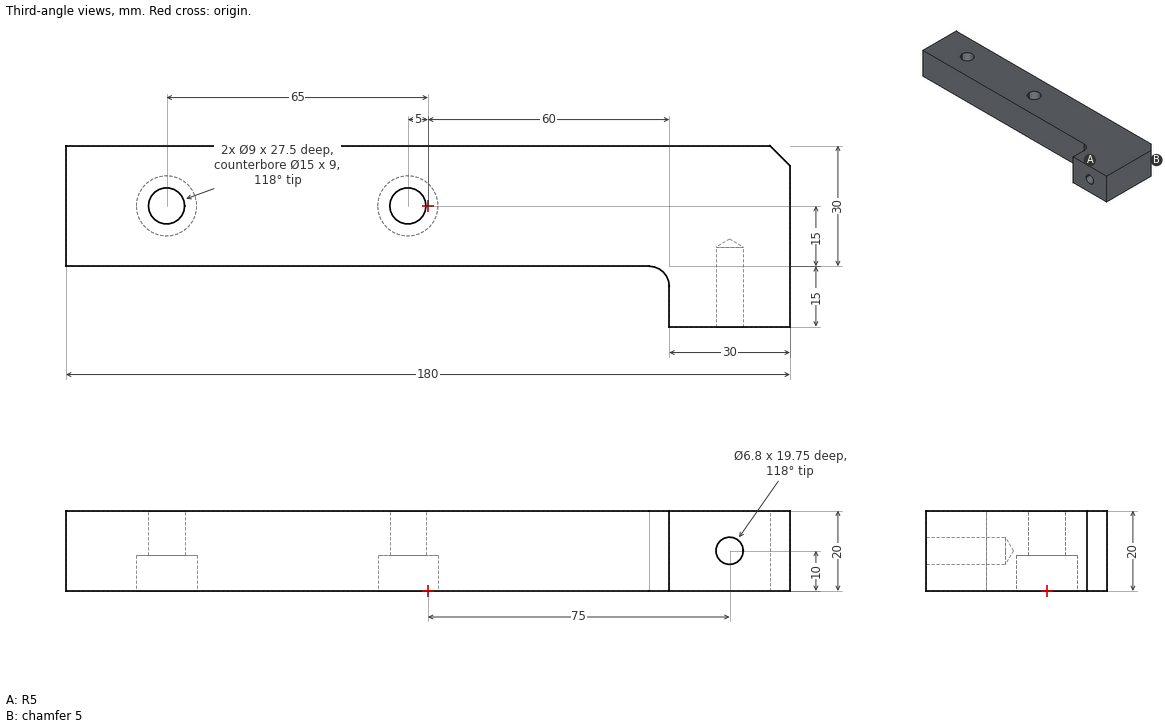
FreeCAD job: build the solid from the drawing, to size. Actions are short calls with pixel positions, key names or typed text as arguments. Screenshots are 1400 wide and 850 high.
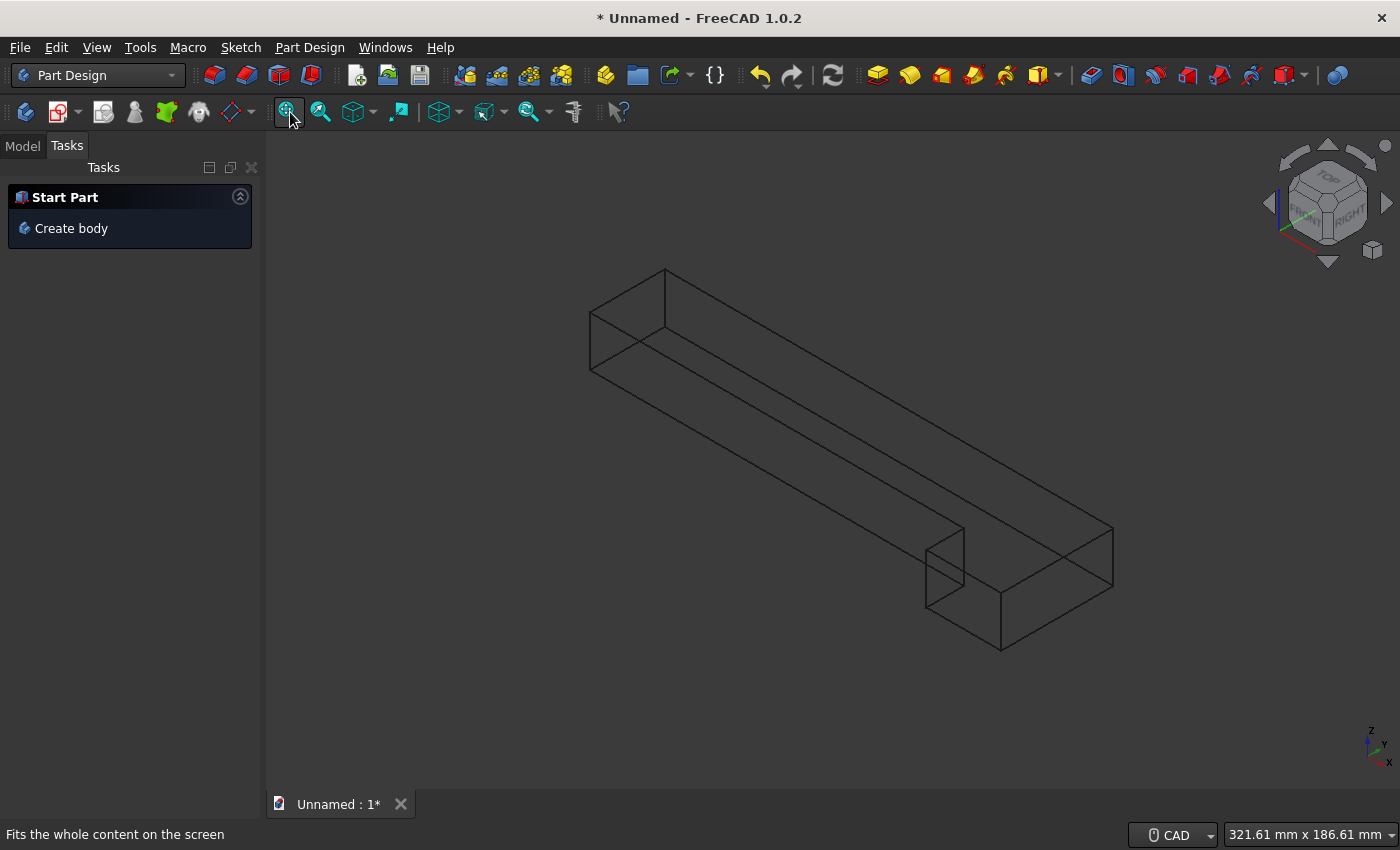
click(964, 556)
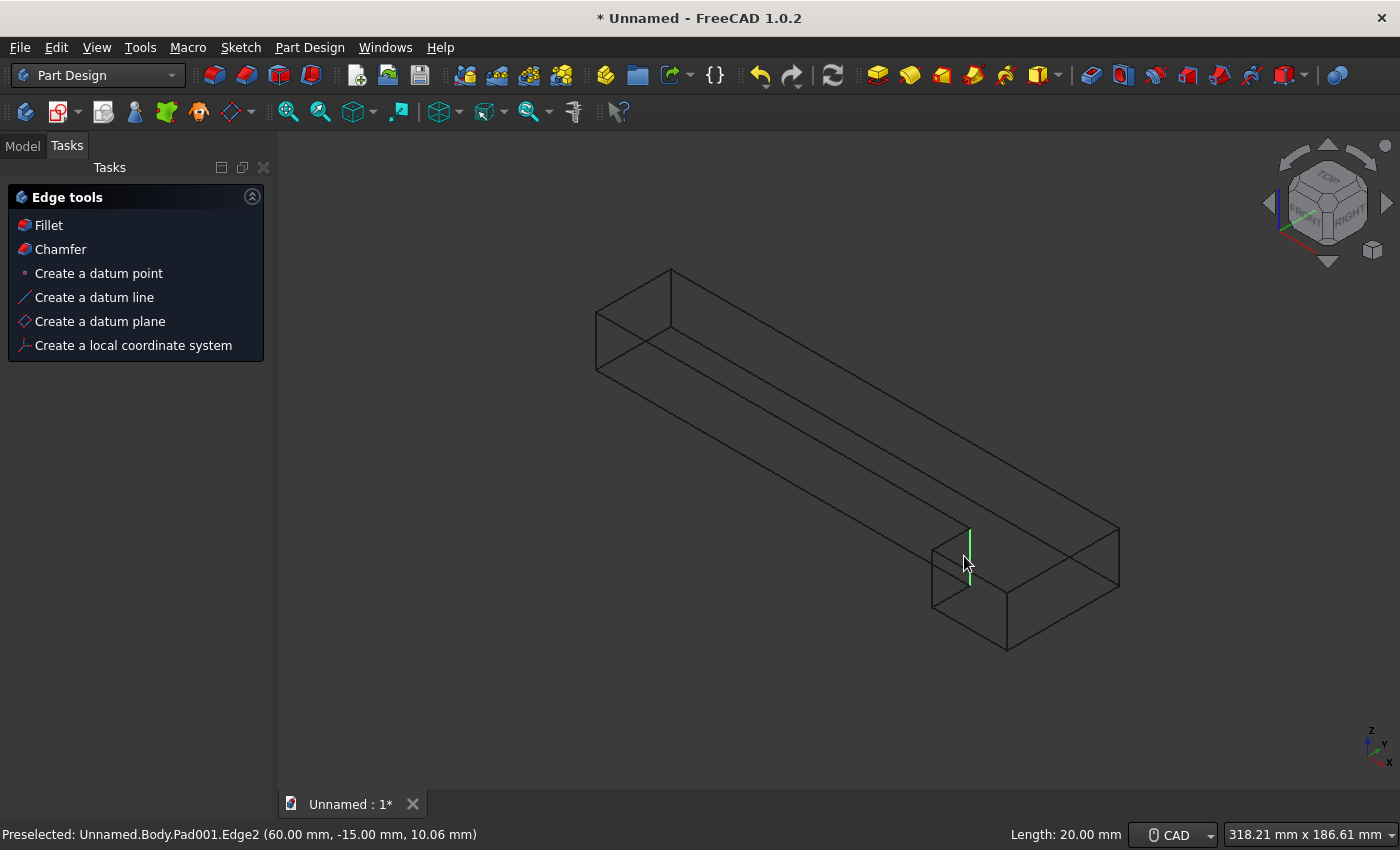
key(v)
key(1)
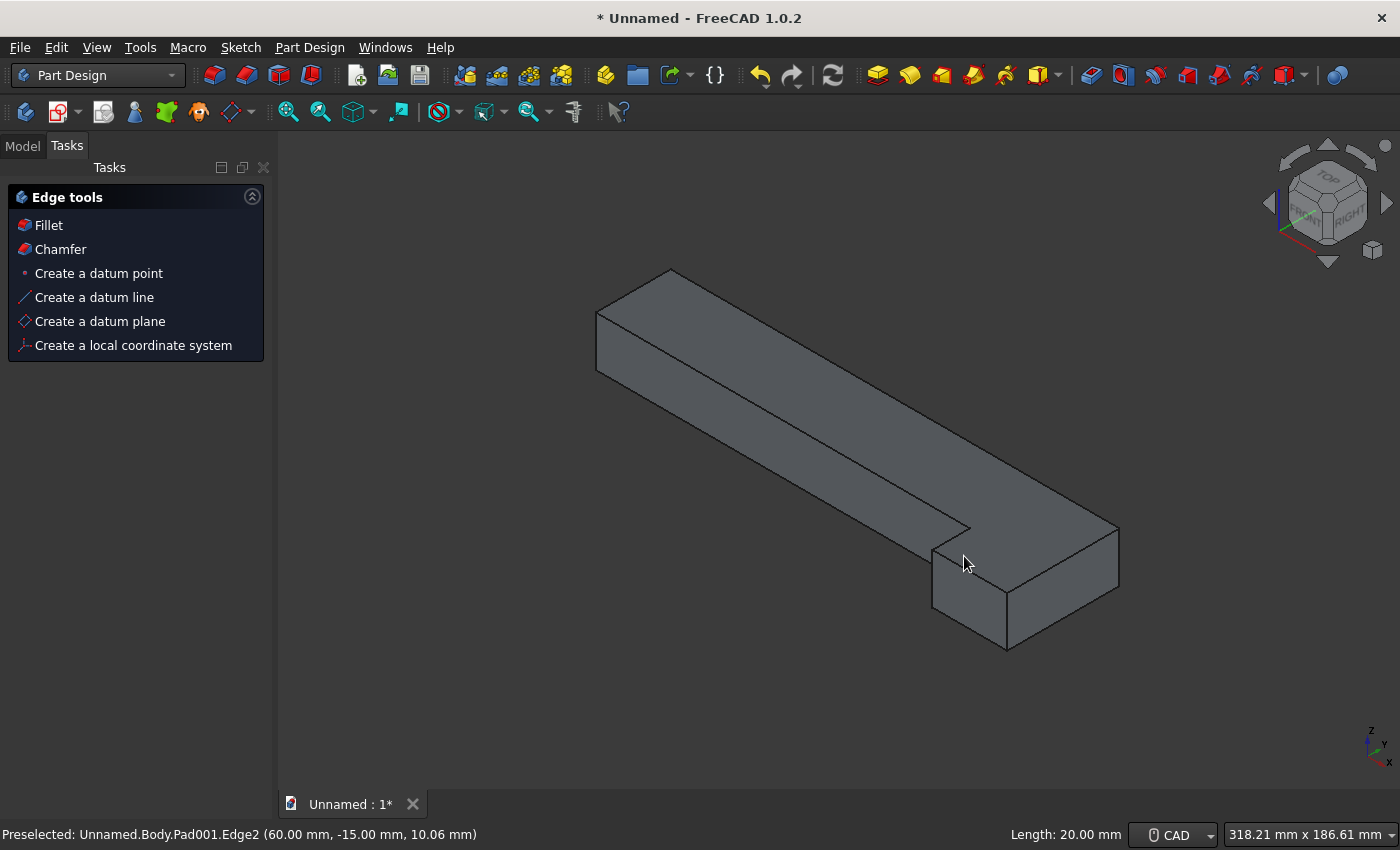
click(216, 76)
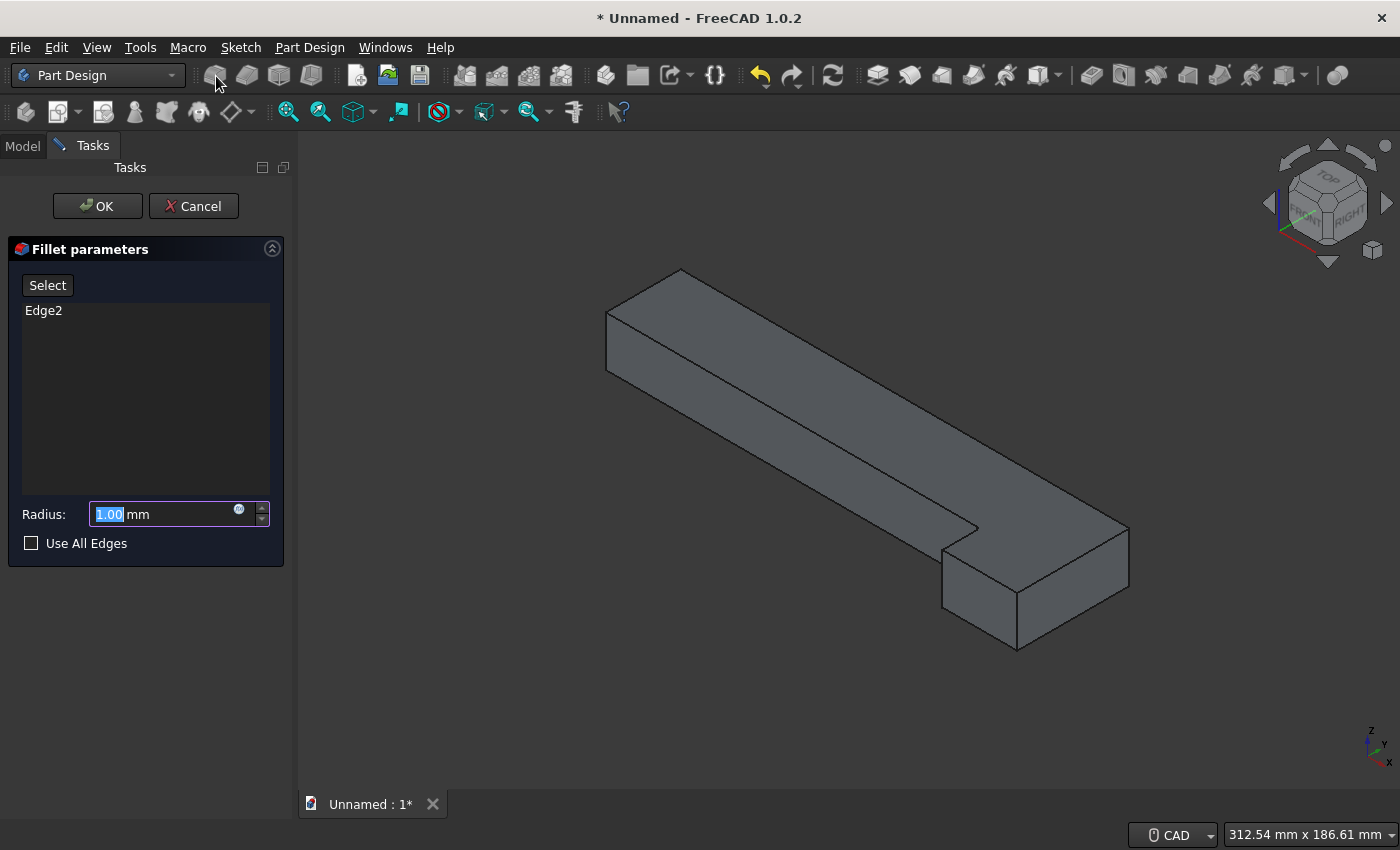
text(5)
key(Tab)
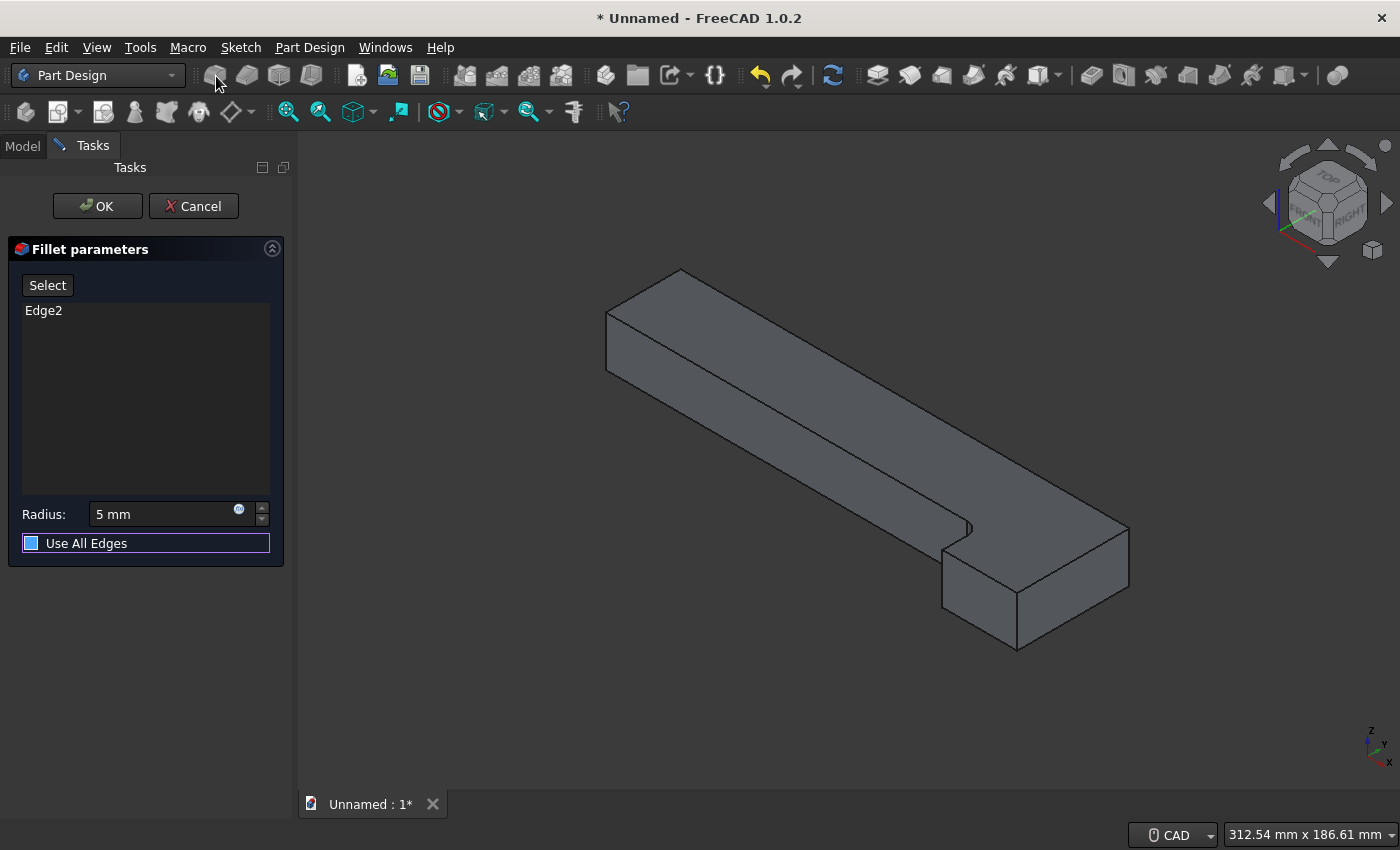
click(98, 206)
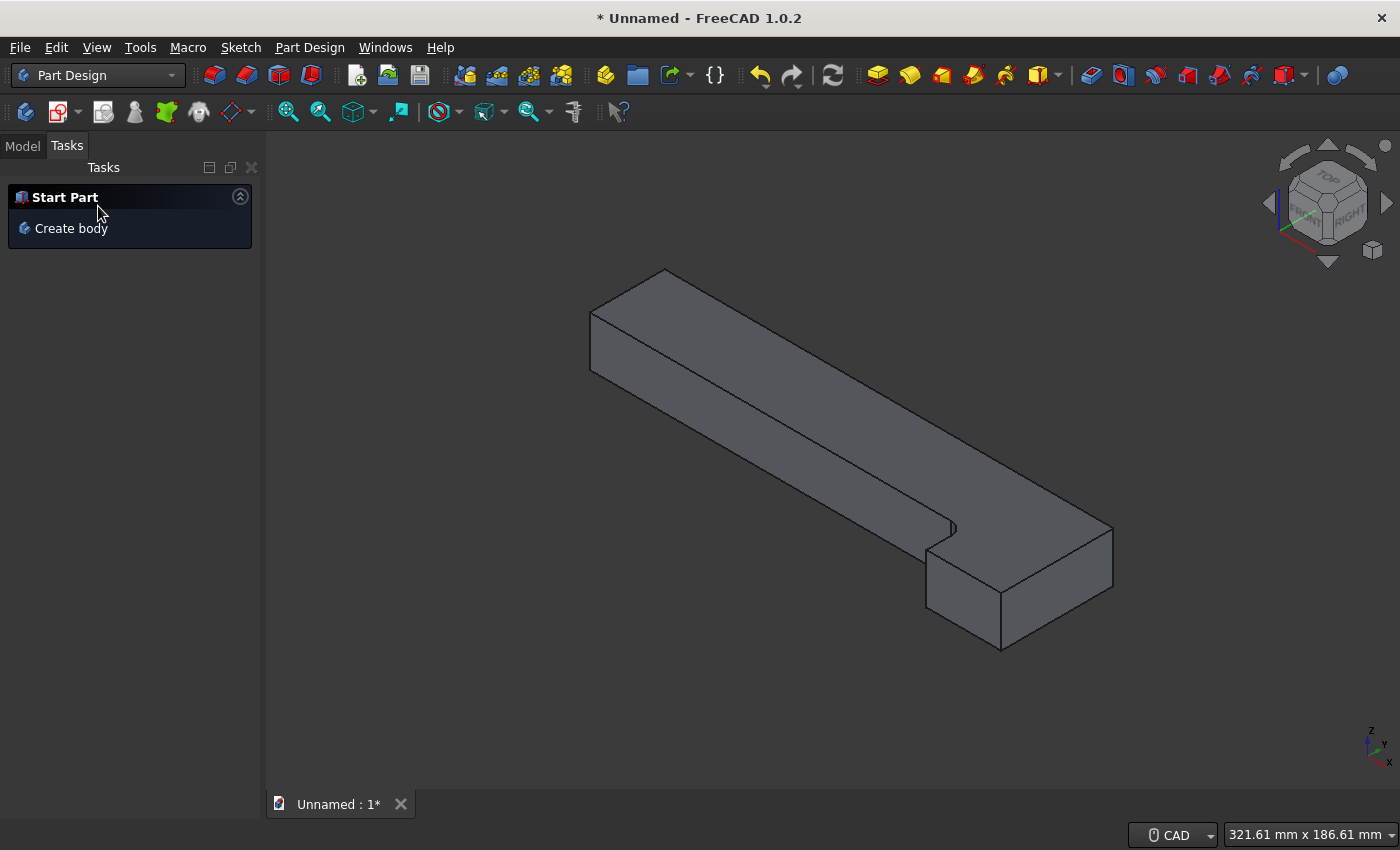
key(2)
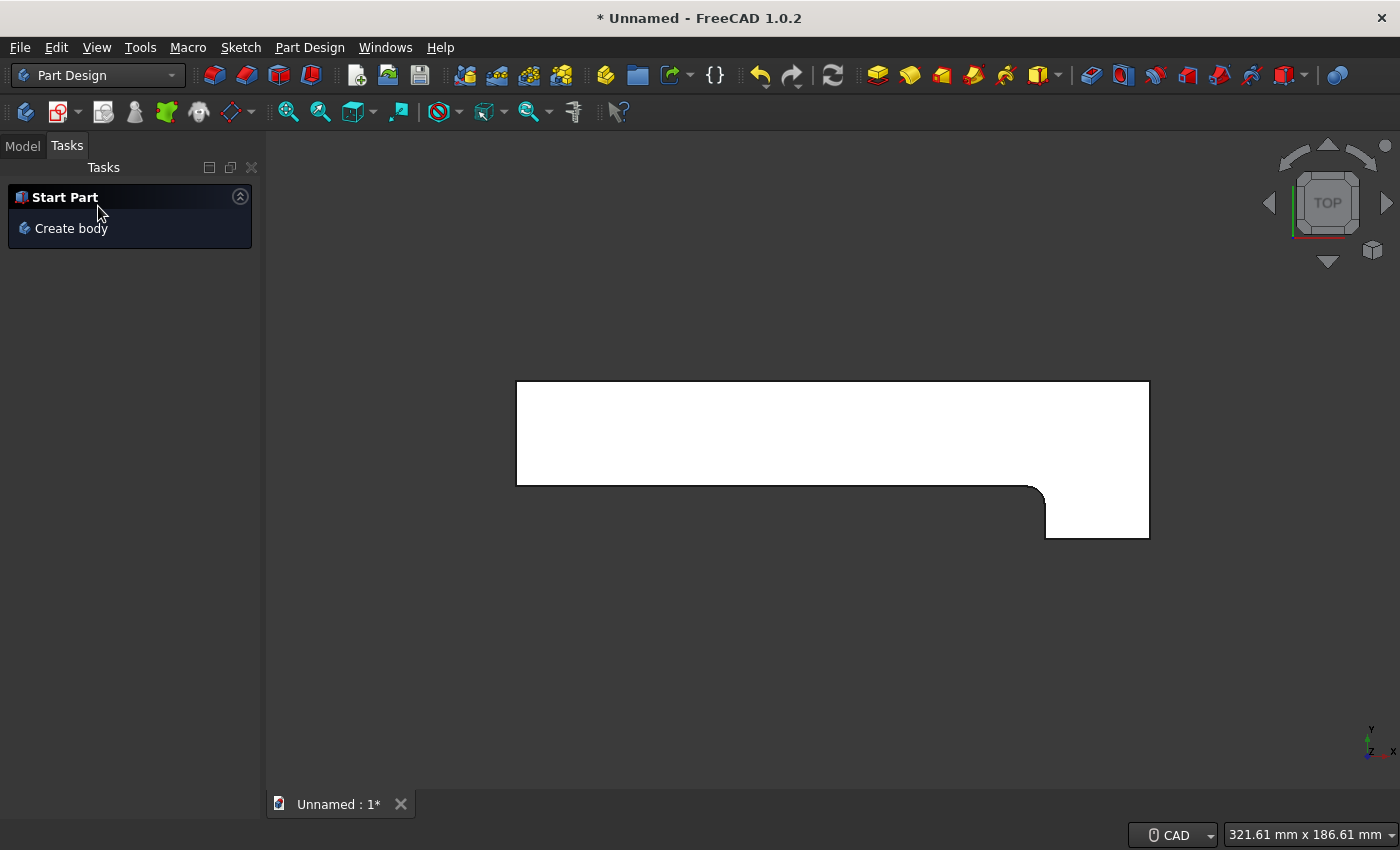
key(0)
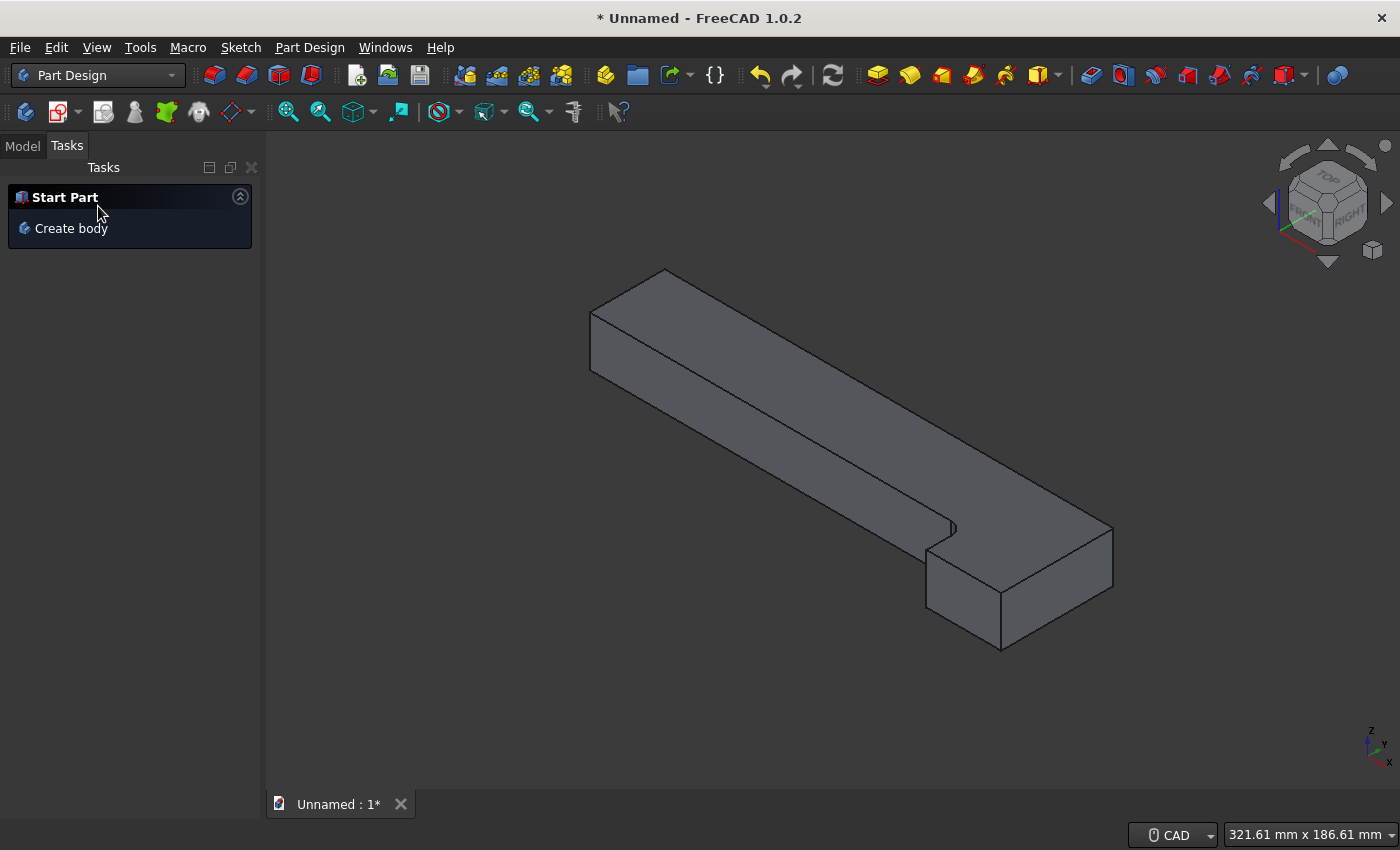
key(1)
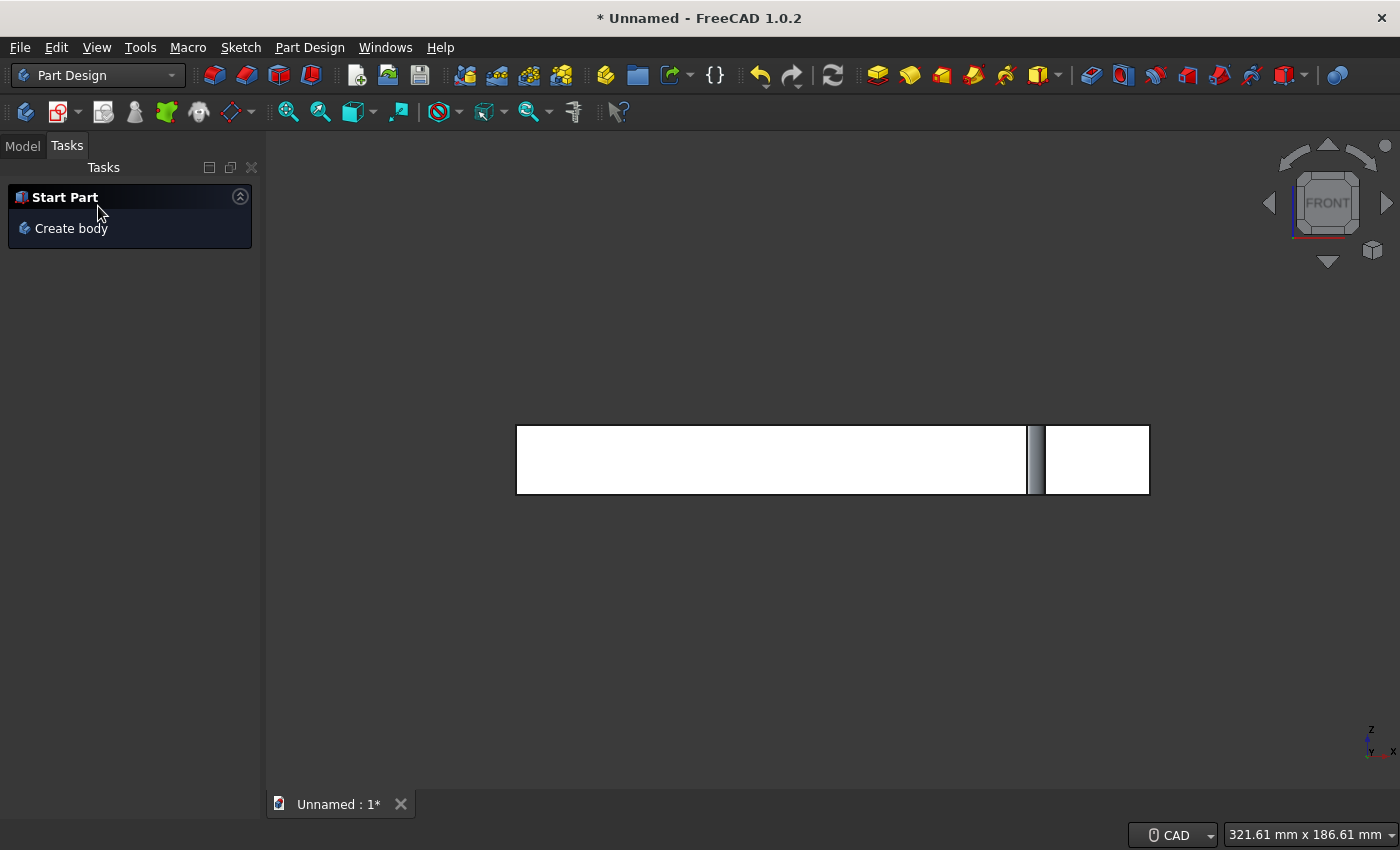
key(3)